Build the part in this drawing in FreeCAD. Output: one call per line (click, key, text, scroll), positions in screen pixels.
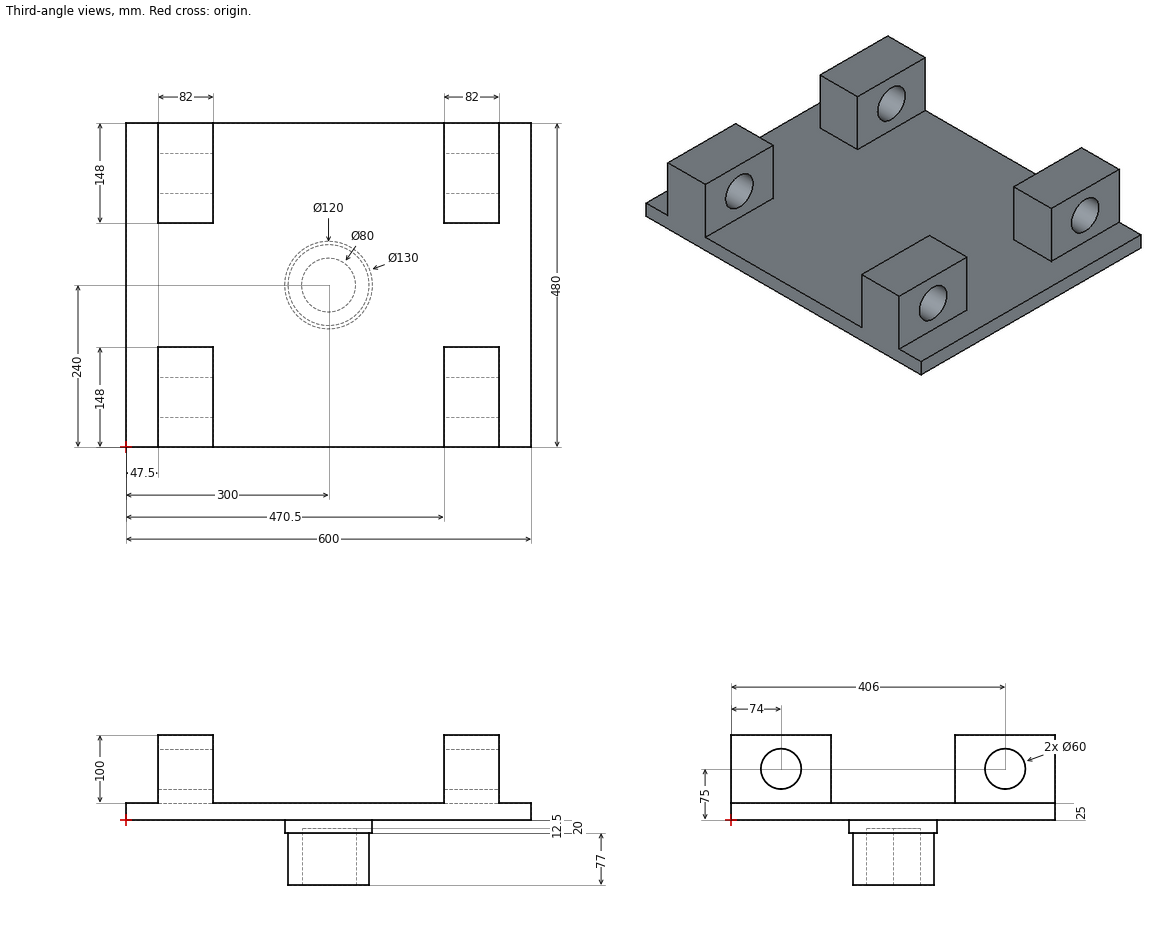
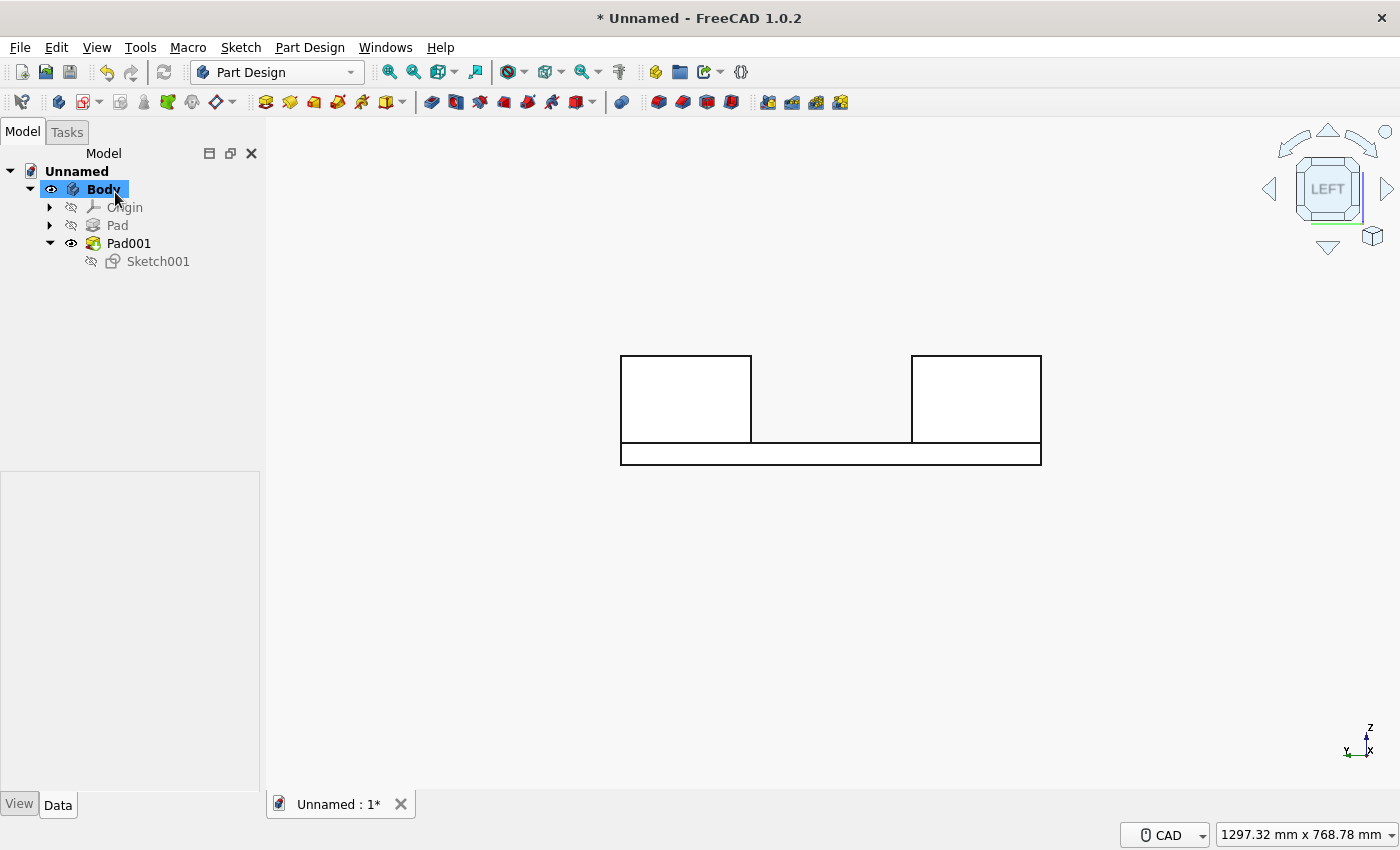
click(390, 72)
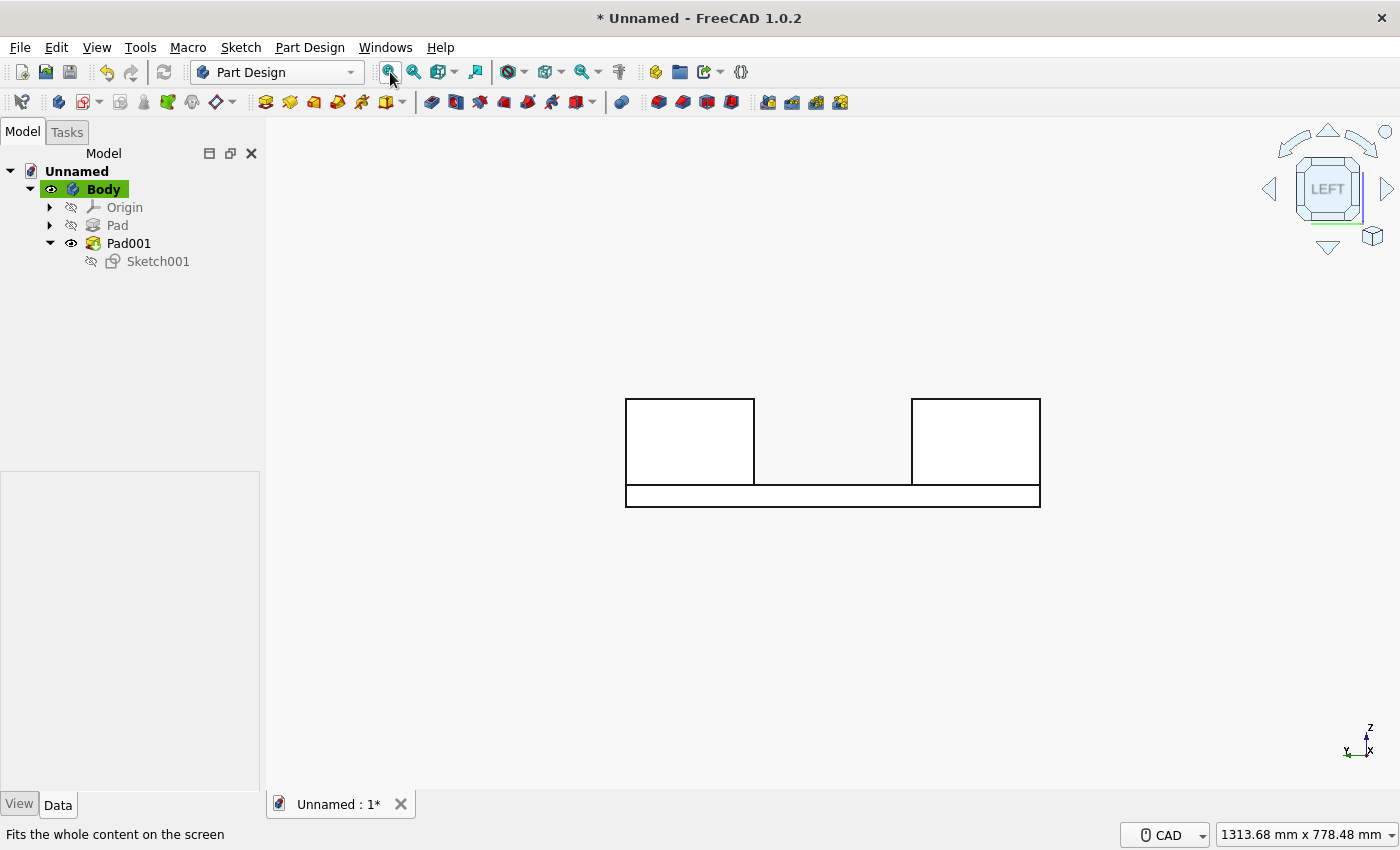
click(671, 441)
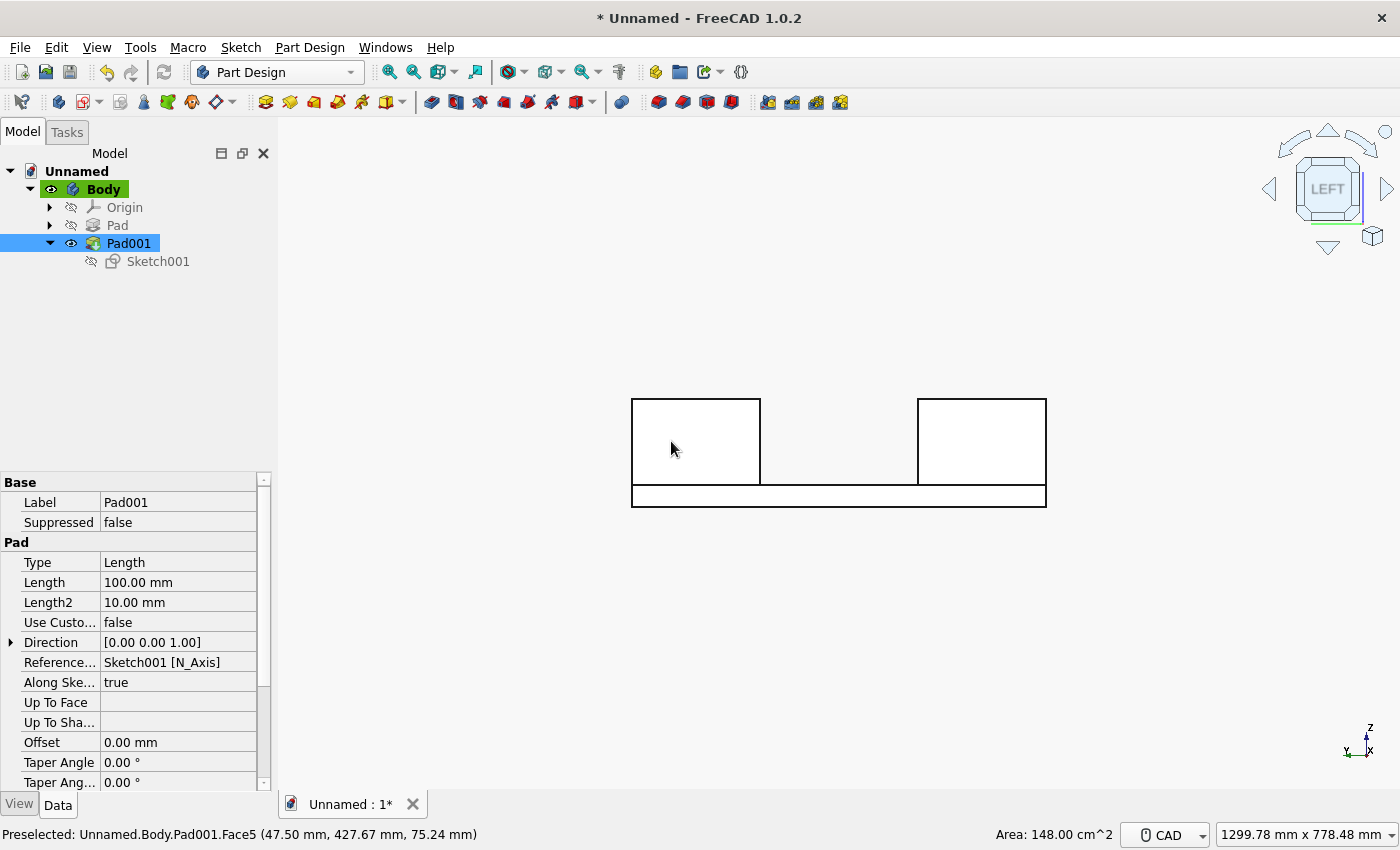
click(84, 102)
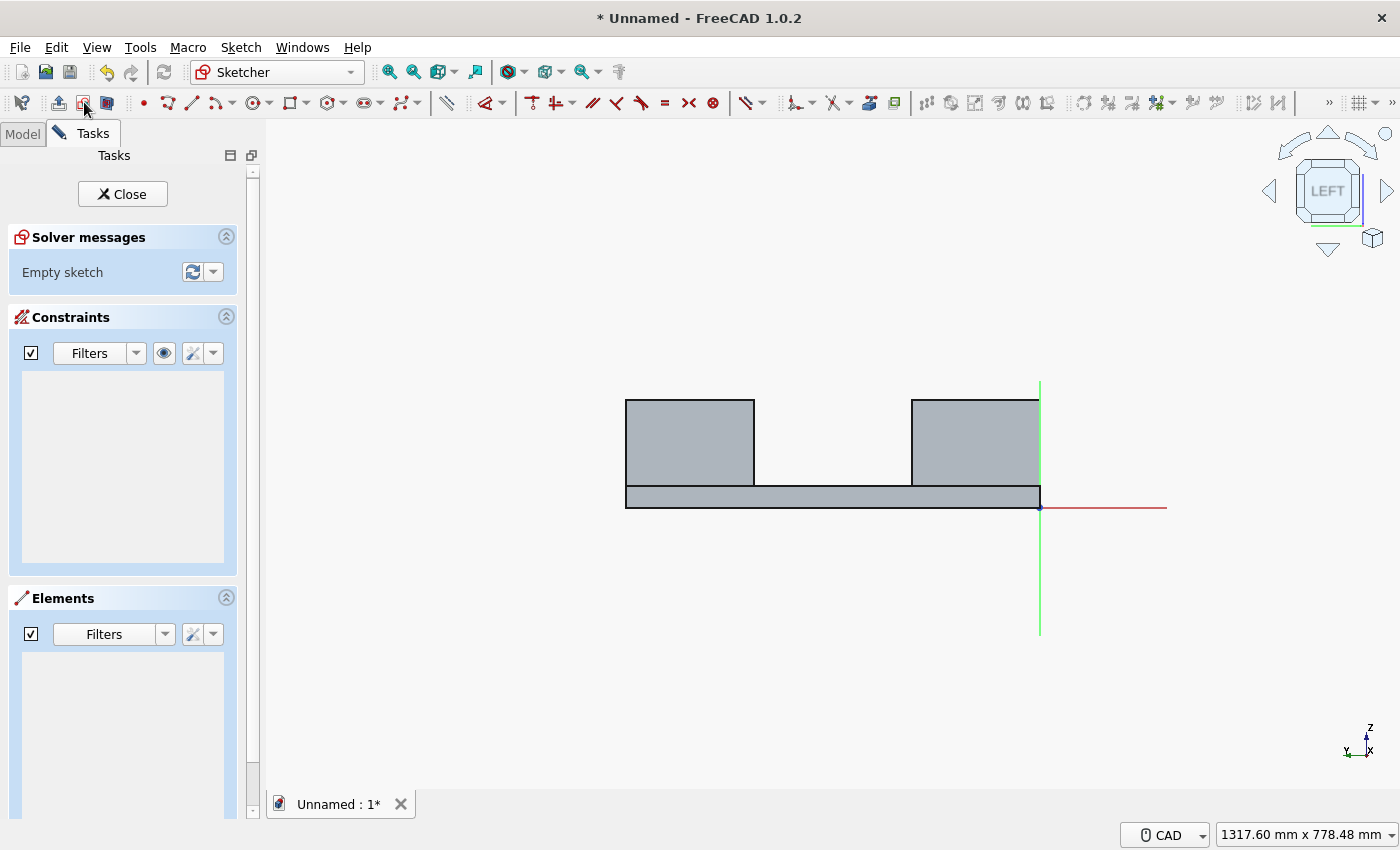
click(108, 104)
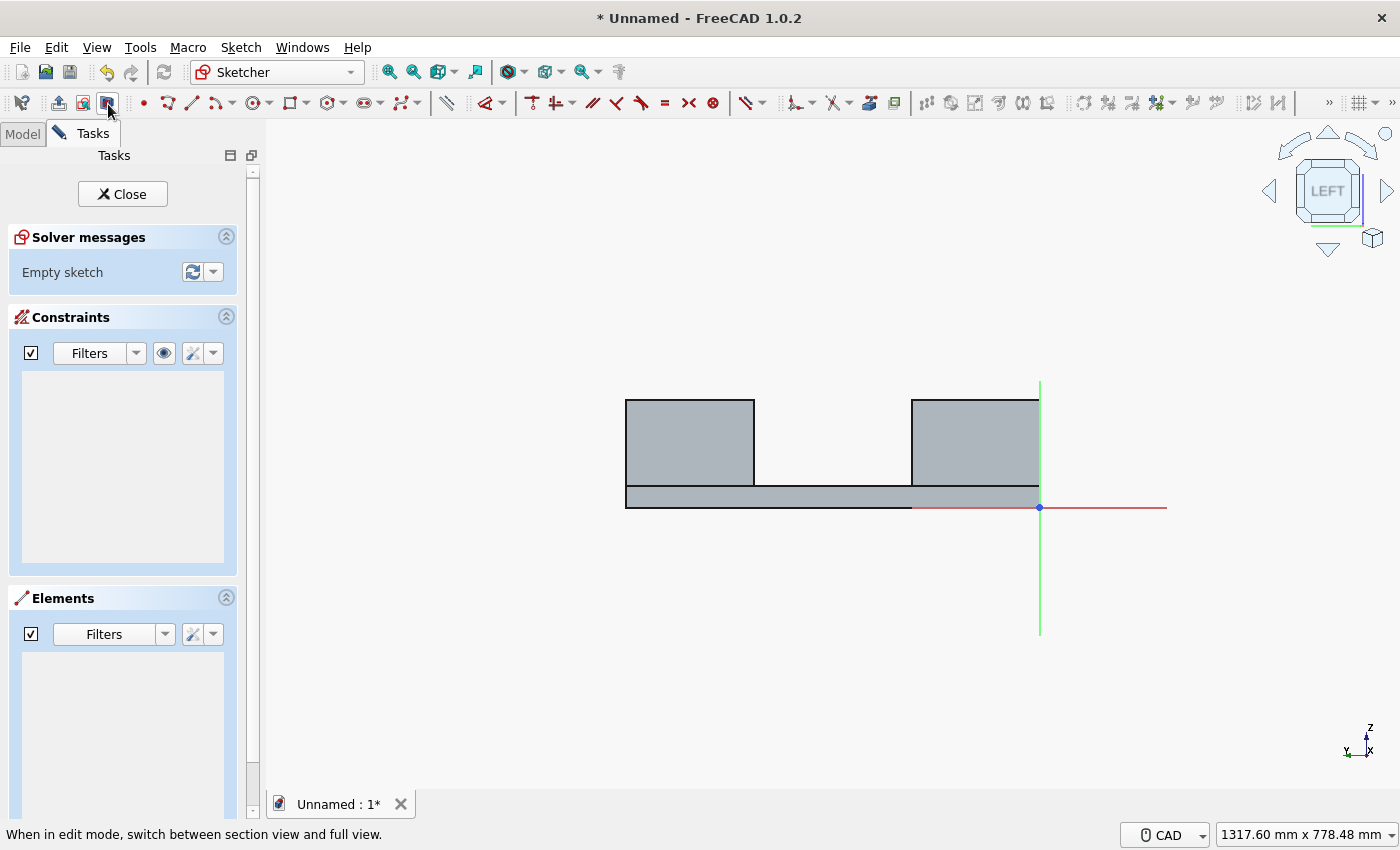
scroll(958, 473, up, 3)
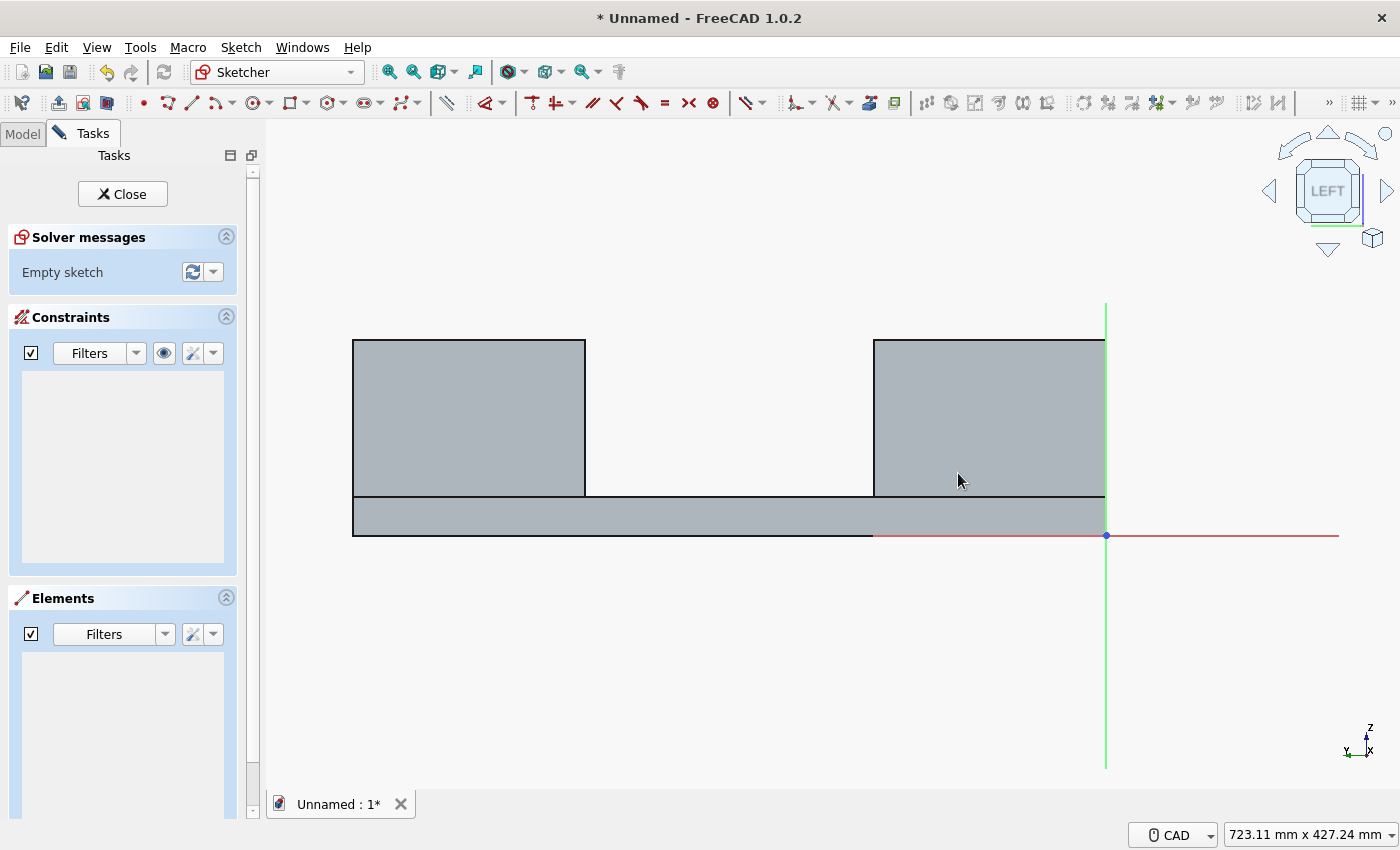
click(254, 104)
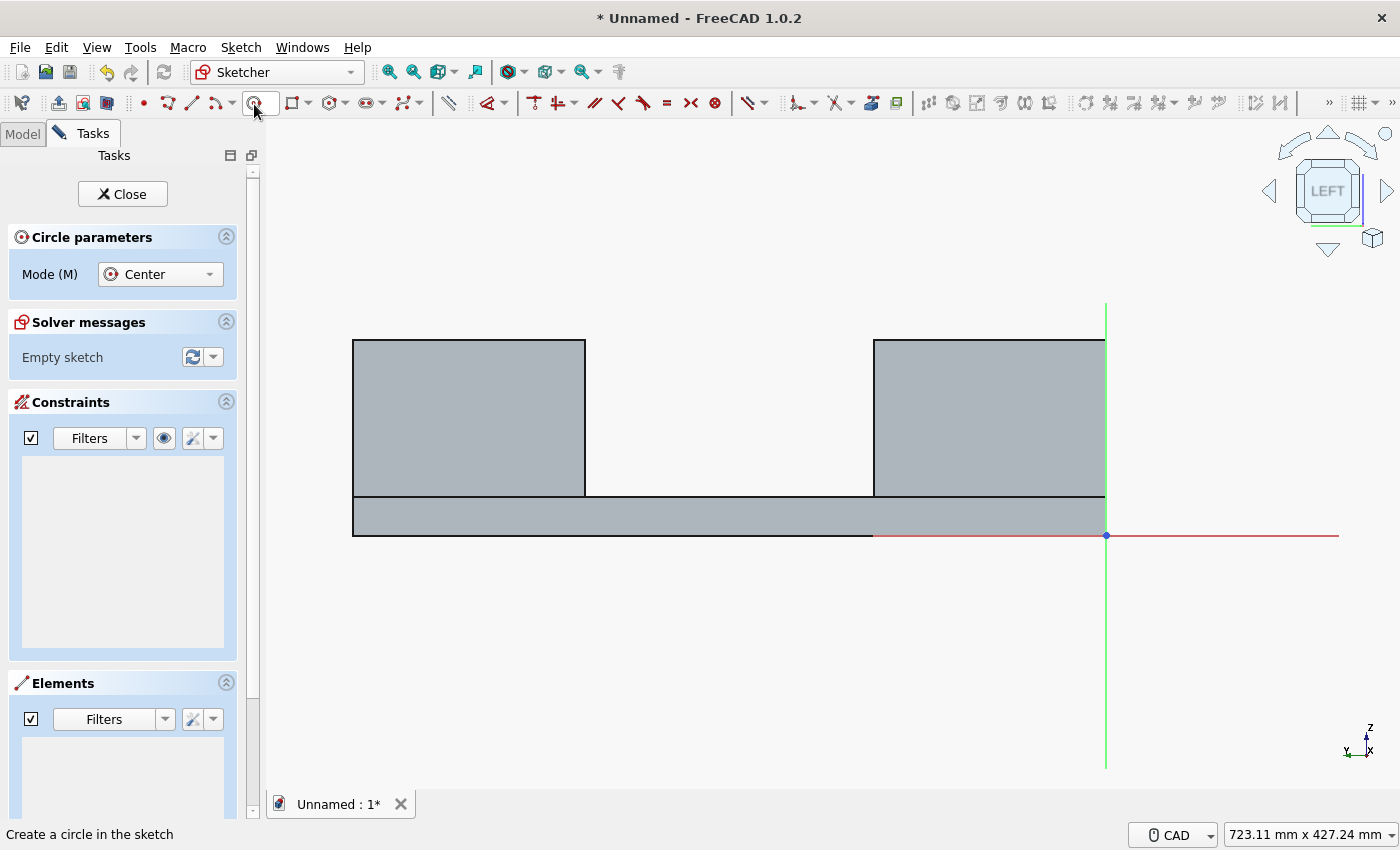
click(469, 418)
move(503, 385)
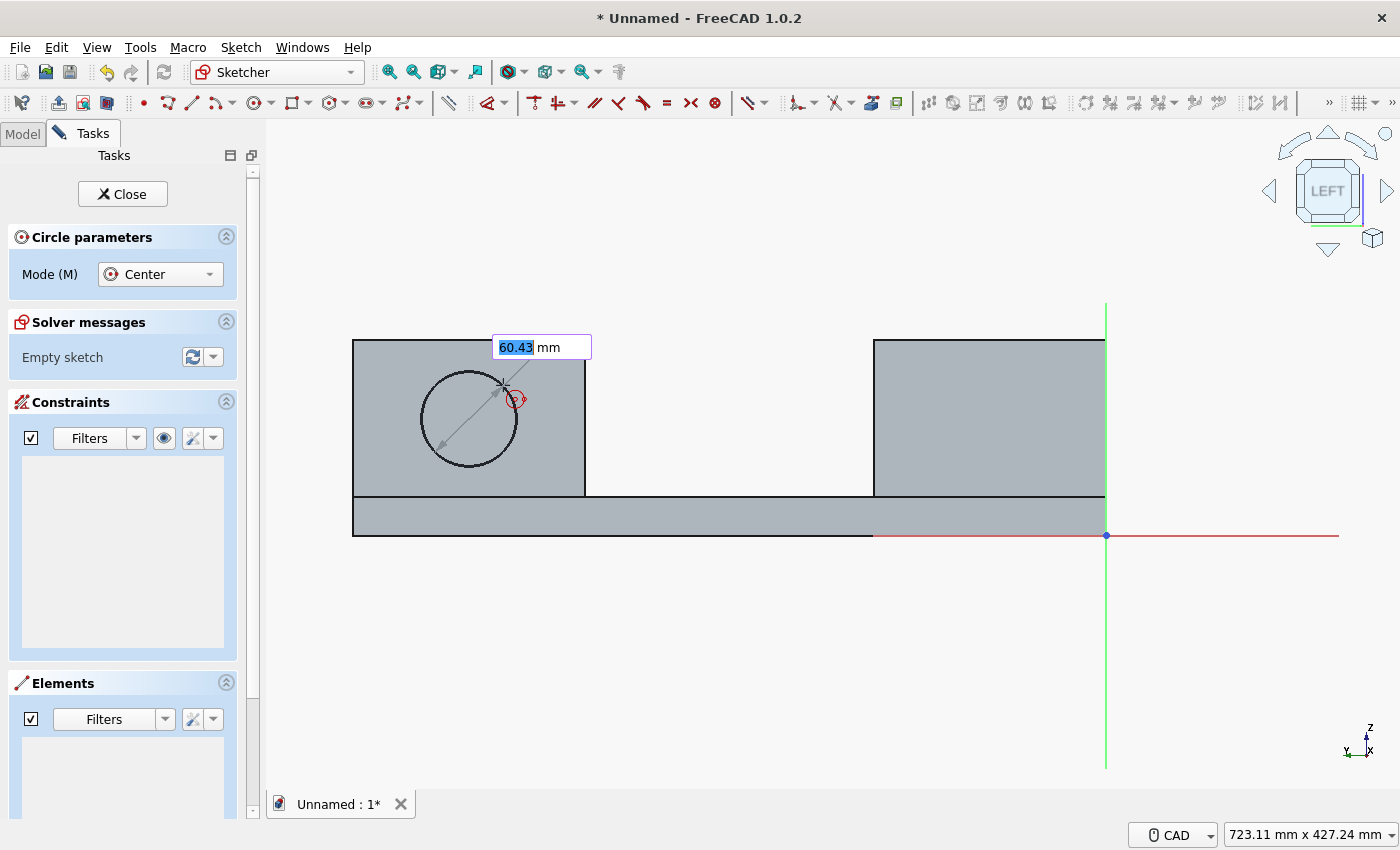
text(60)
key(Return)